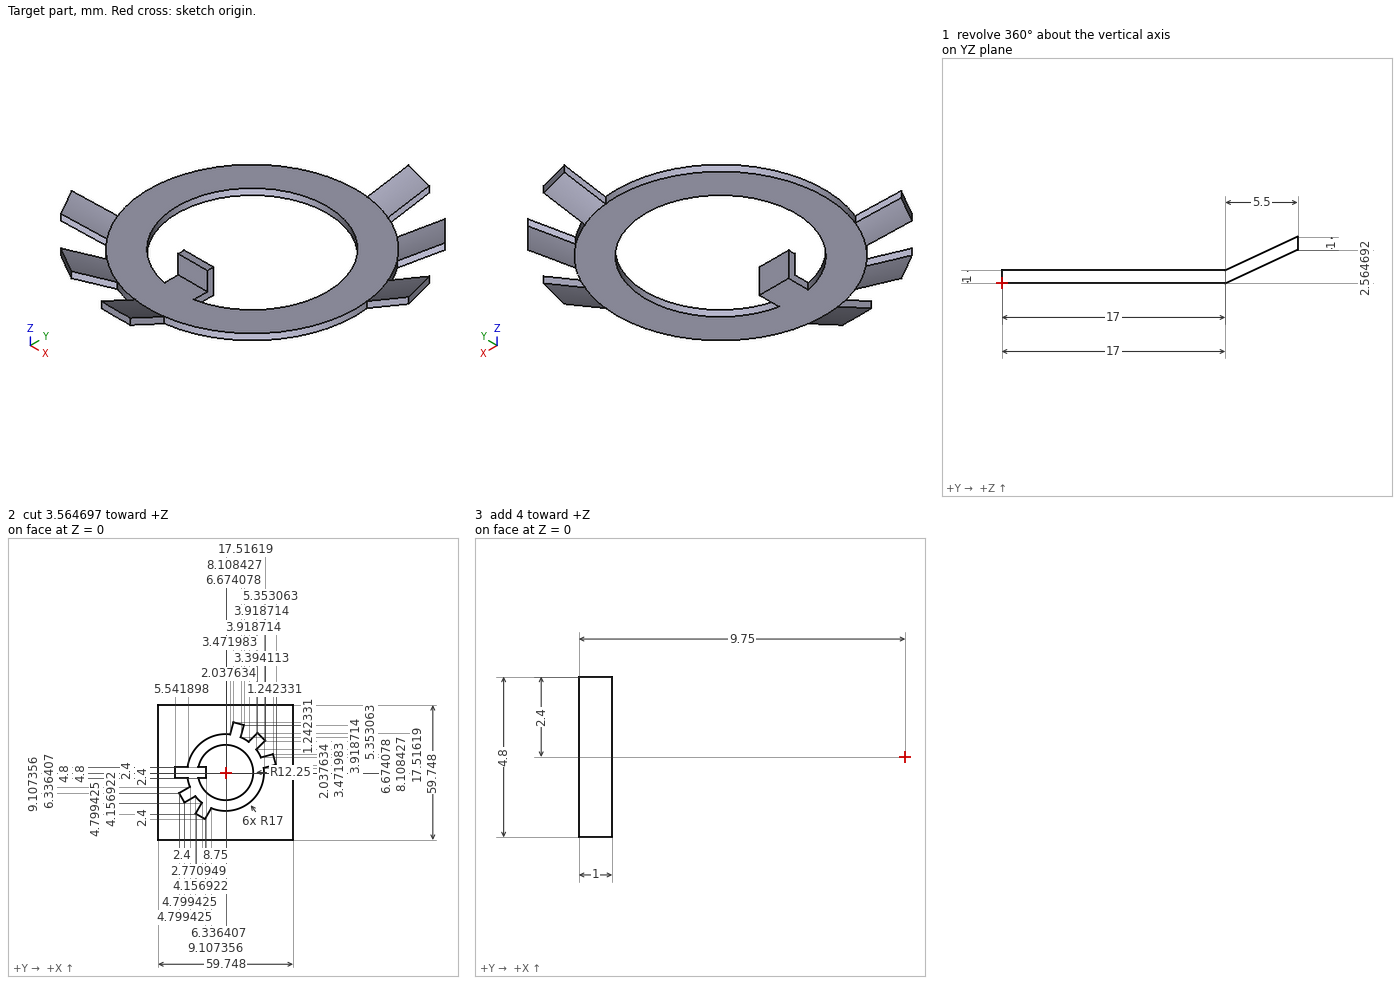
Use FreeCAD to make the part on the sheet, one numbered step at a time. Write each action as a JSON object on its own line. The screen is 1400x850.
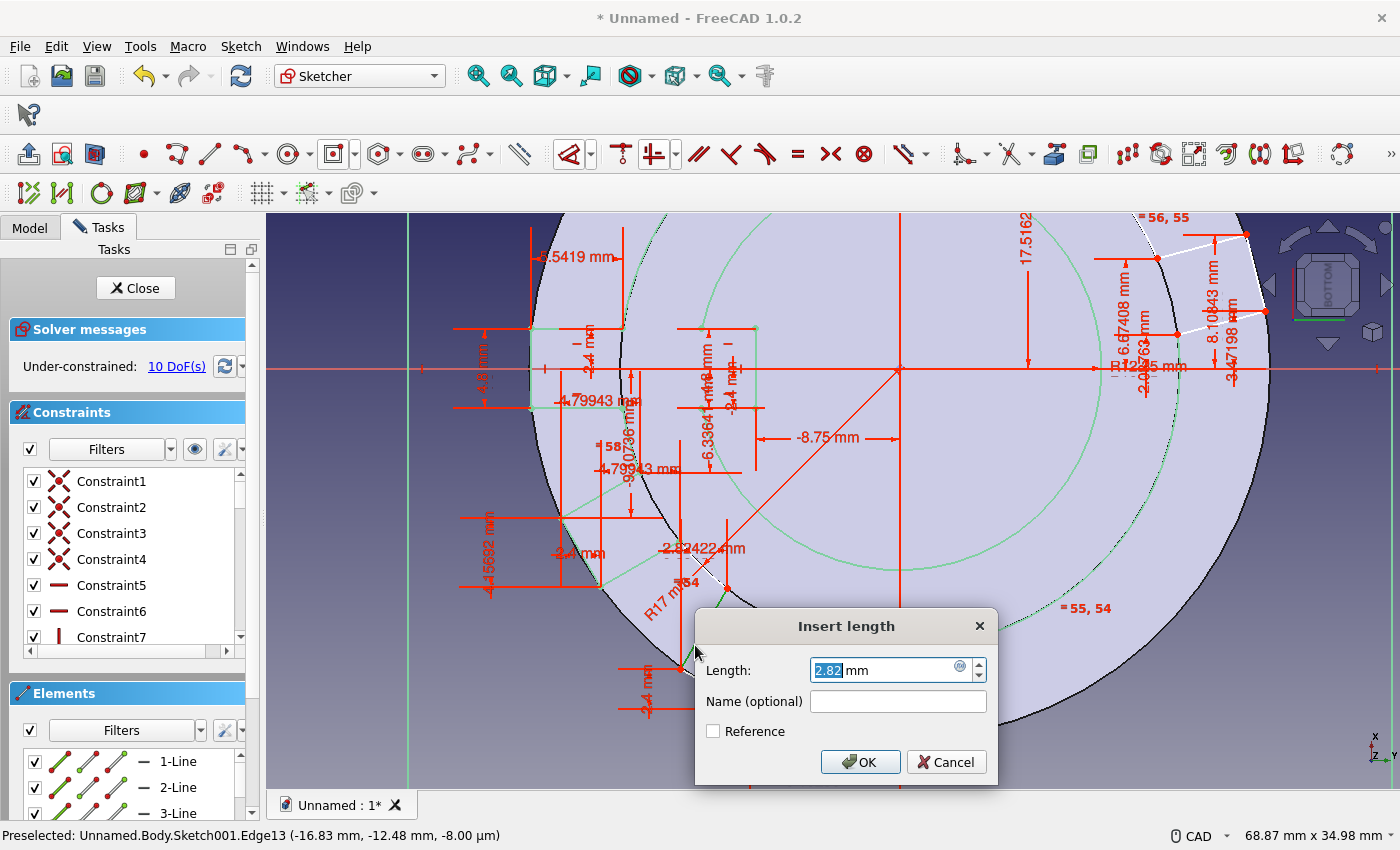
{"action": "type", "text": "2.770949"}
{"action": "key", "text": "Return"}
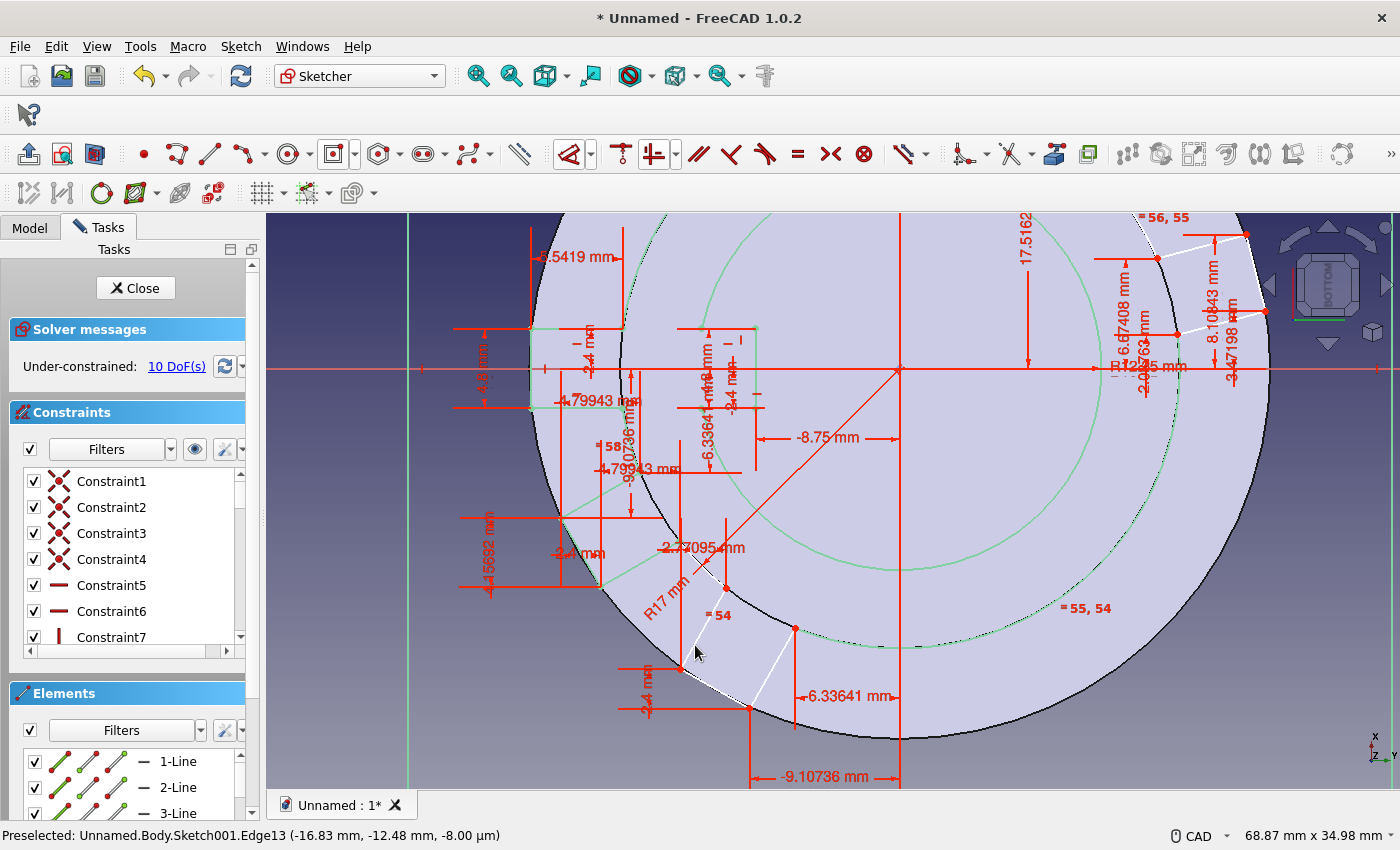
{"action": "left_click", "coordinate": [694, 645]}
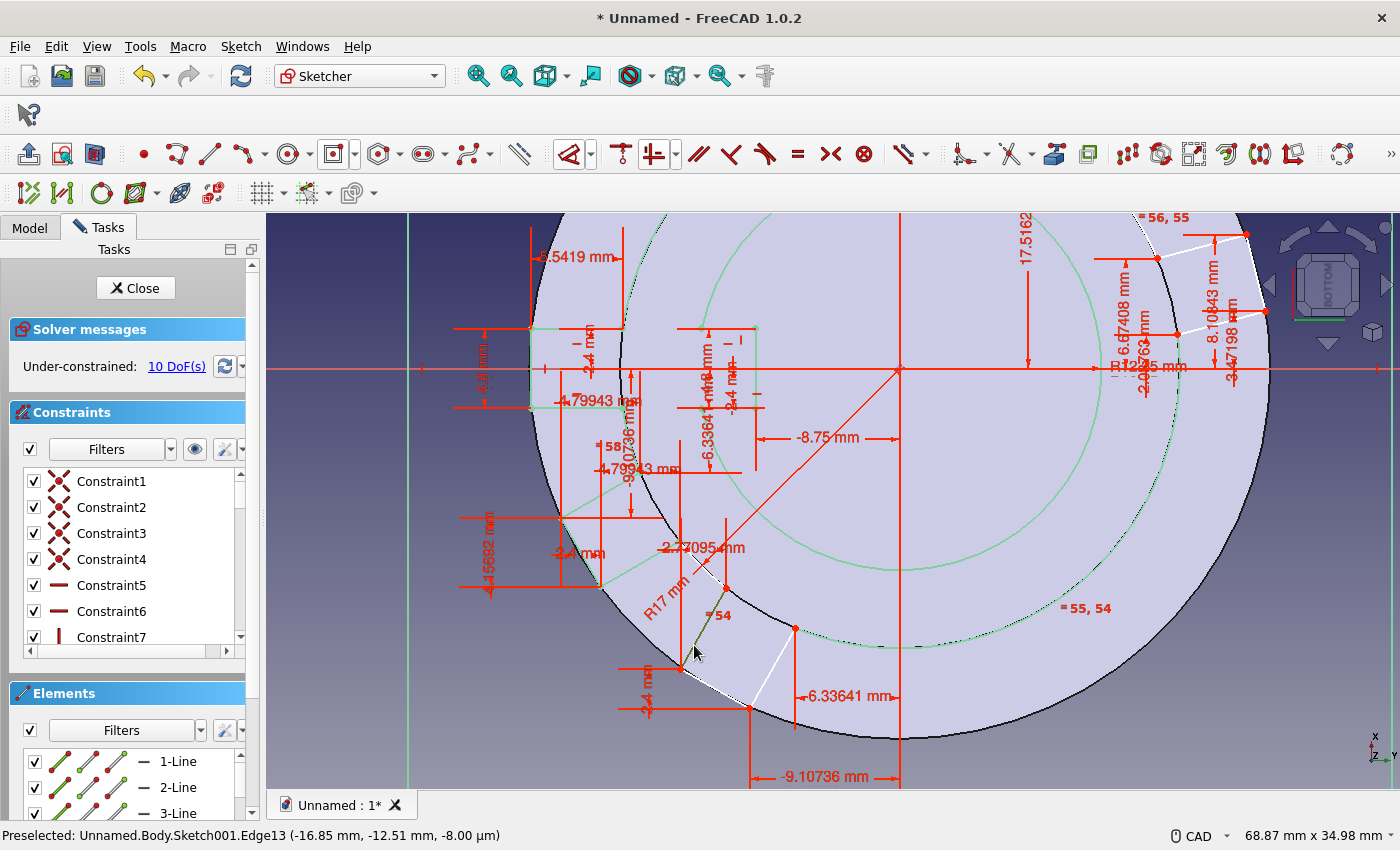
{"action": "key", "text": "i"}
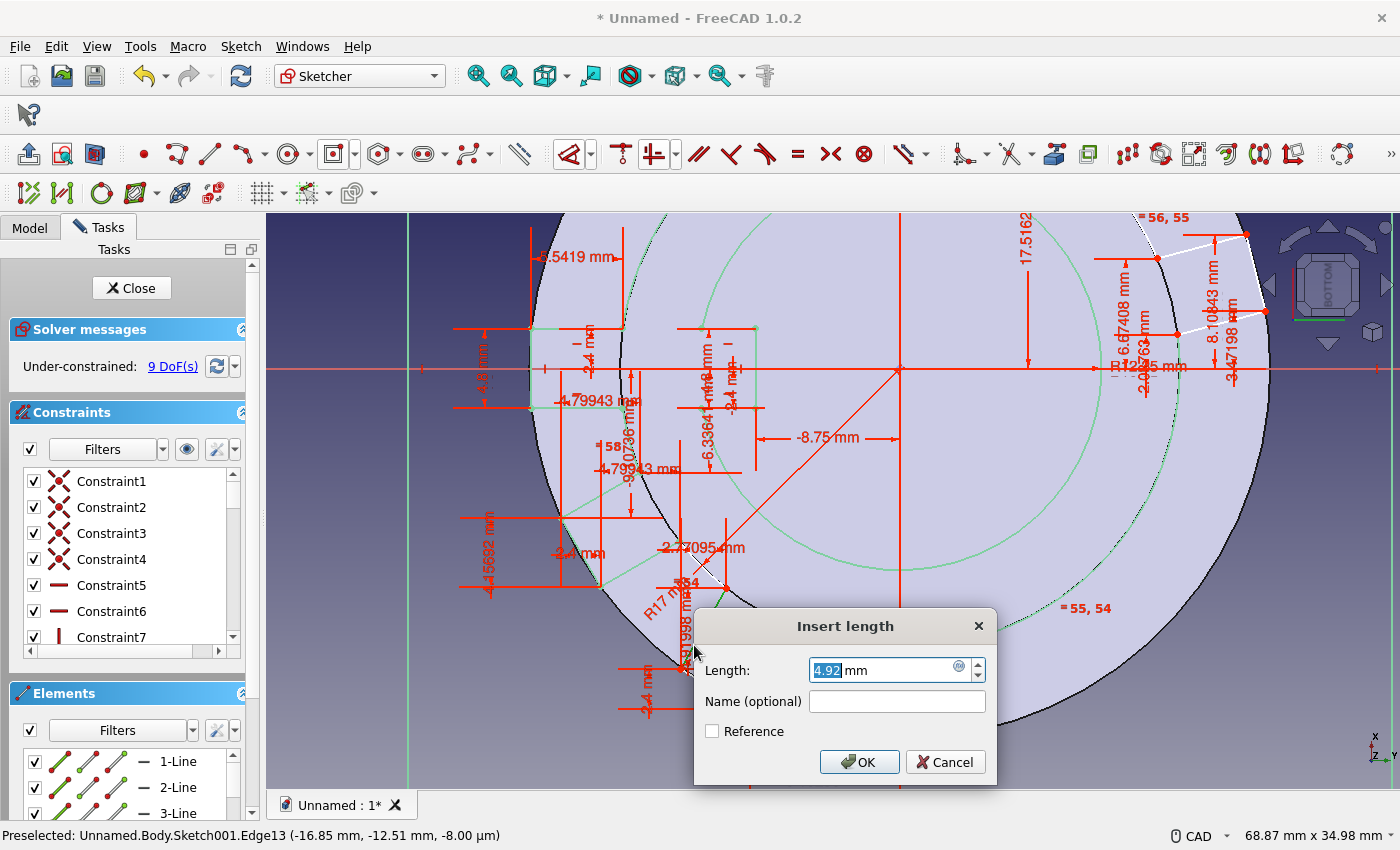
{"action": "type", "text": "4.799425"}
{"action": "key", "text": "Return"}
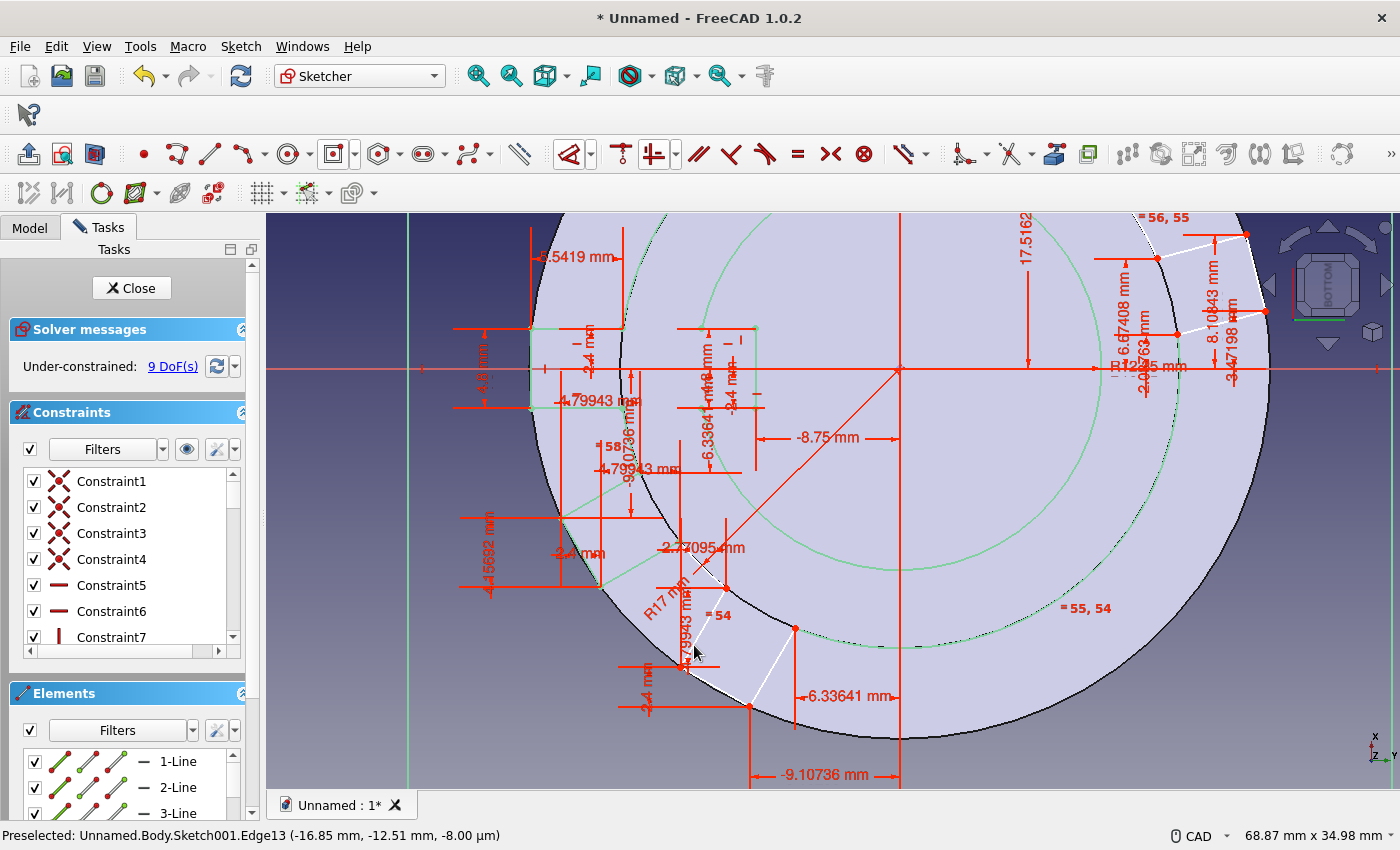
{"action": "left_click", "coordinate": [701, 679]}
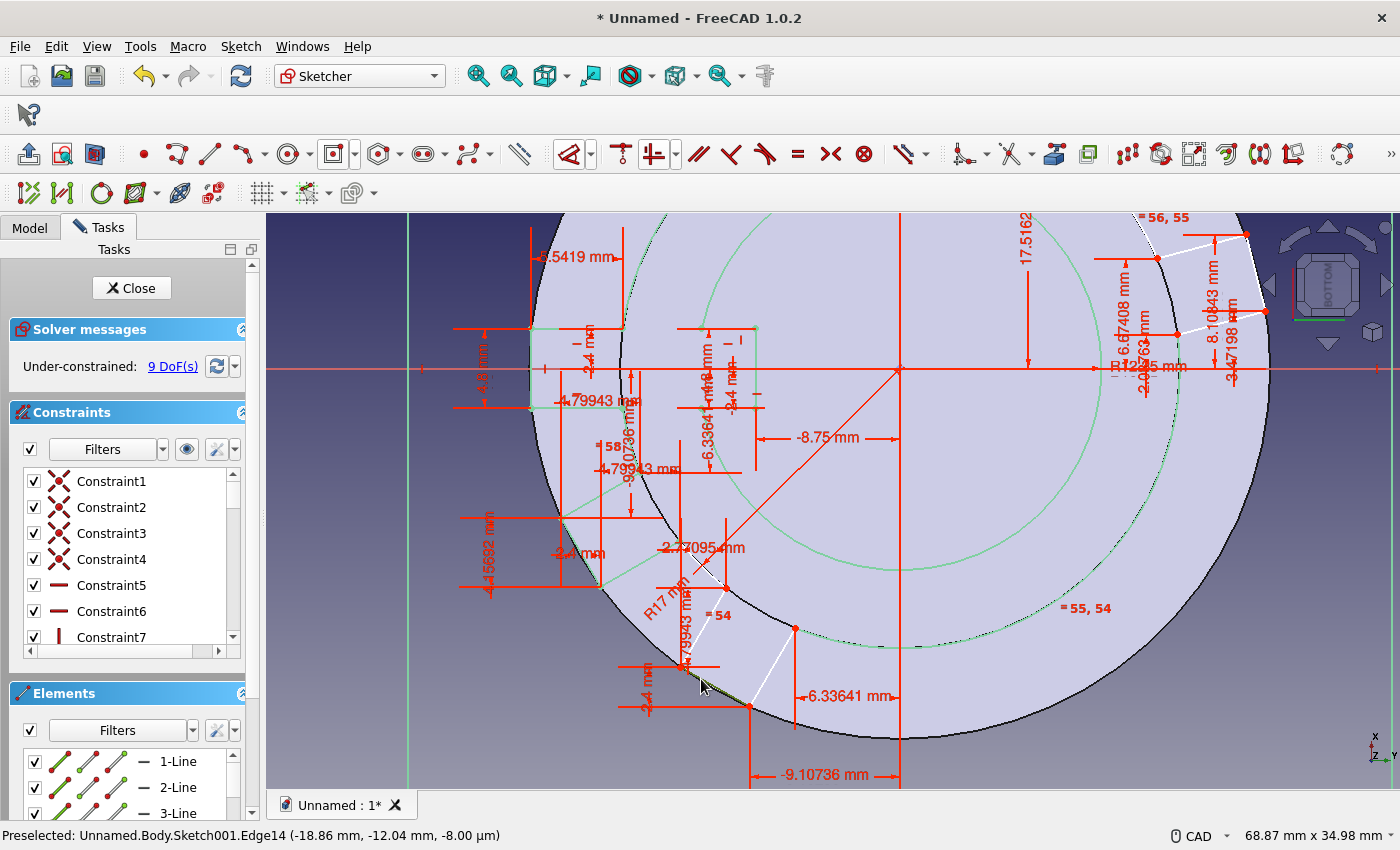
{"action": "left_click", "coordinate": [590, 154]}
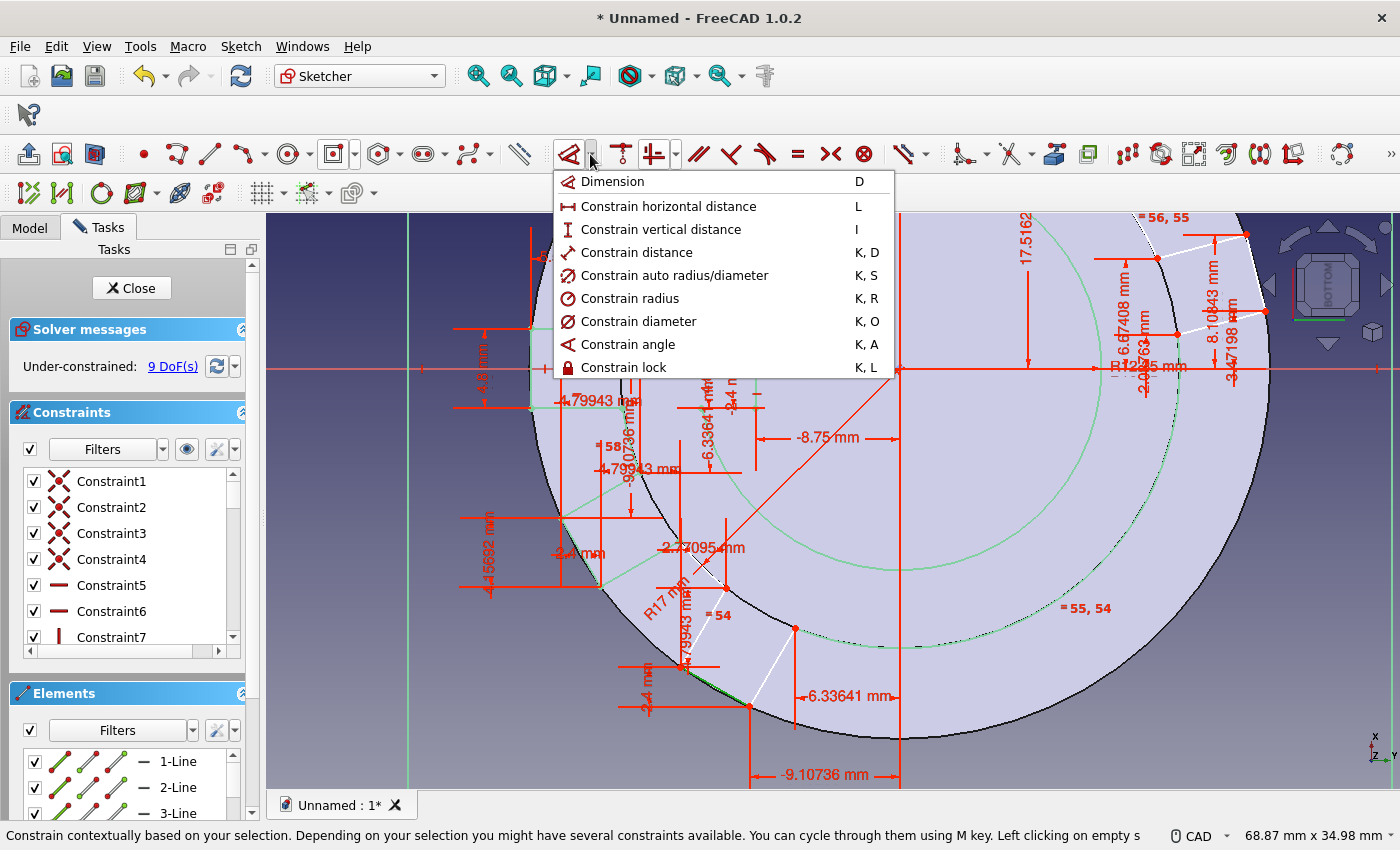
{"action": "left_click", "coordinate": [724, 206]}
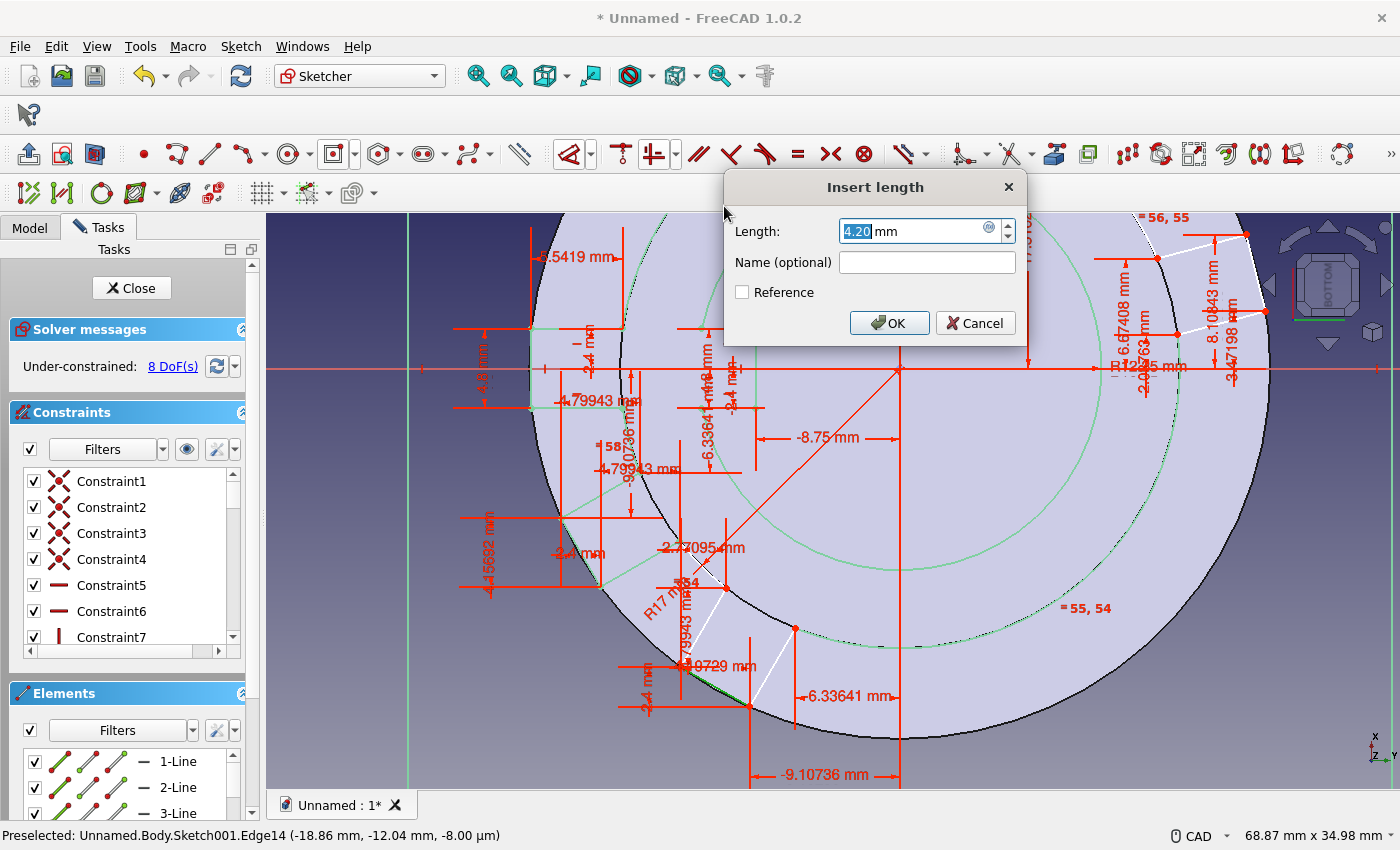
{"action": "type", "text": "4.156922"}
{"action": "key", "text": "Return"}